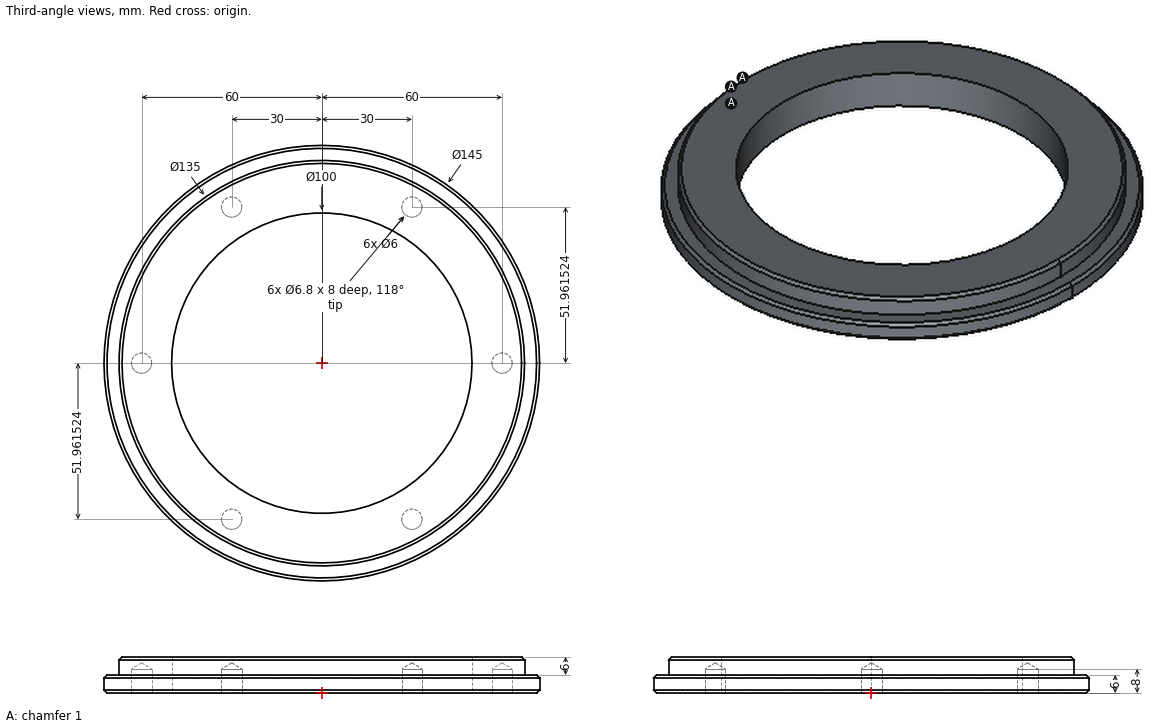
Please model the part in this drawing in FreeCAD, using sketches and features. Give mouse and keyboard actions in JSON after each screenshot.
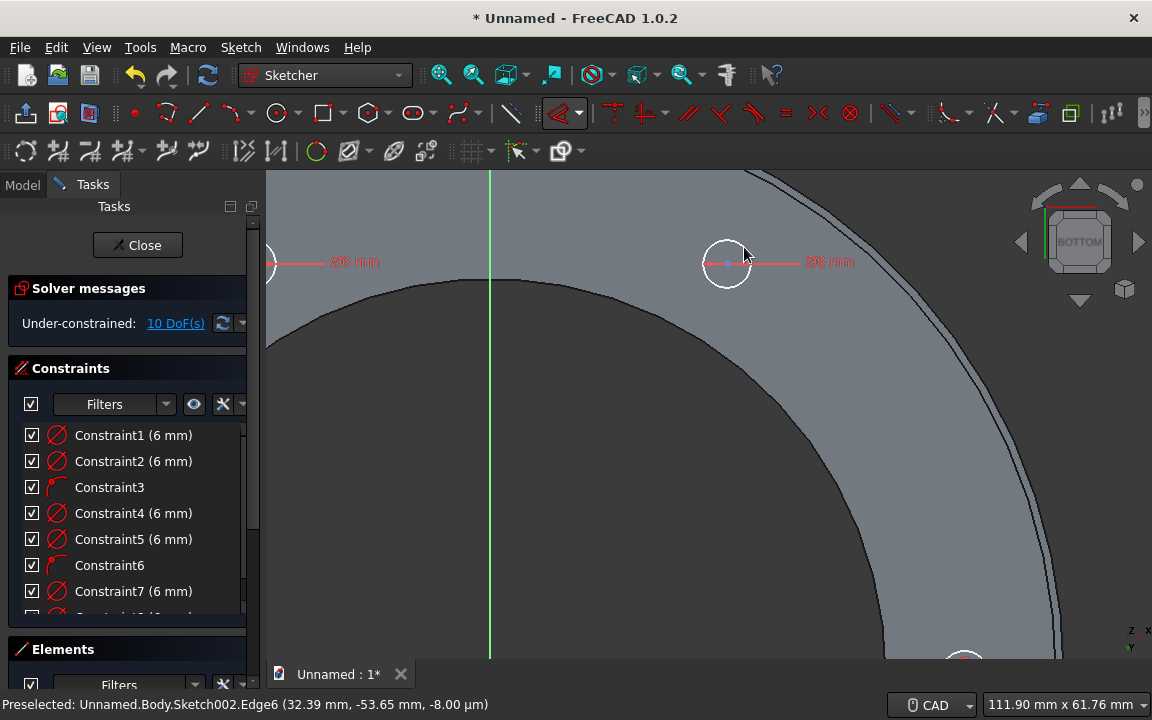
{"action": "scroll", "coordinate": [728, 263], "scroll_direction": "down", "scroll_amount": 5}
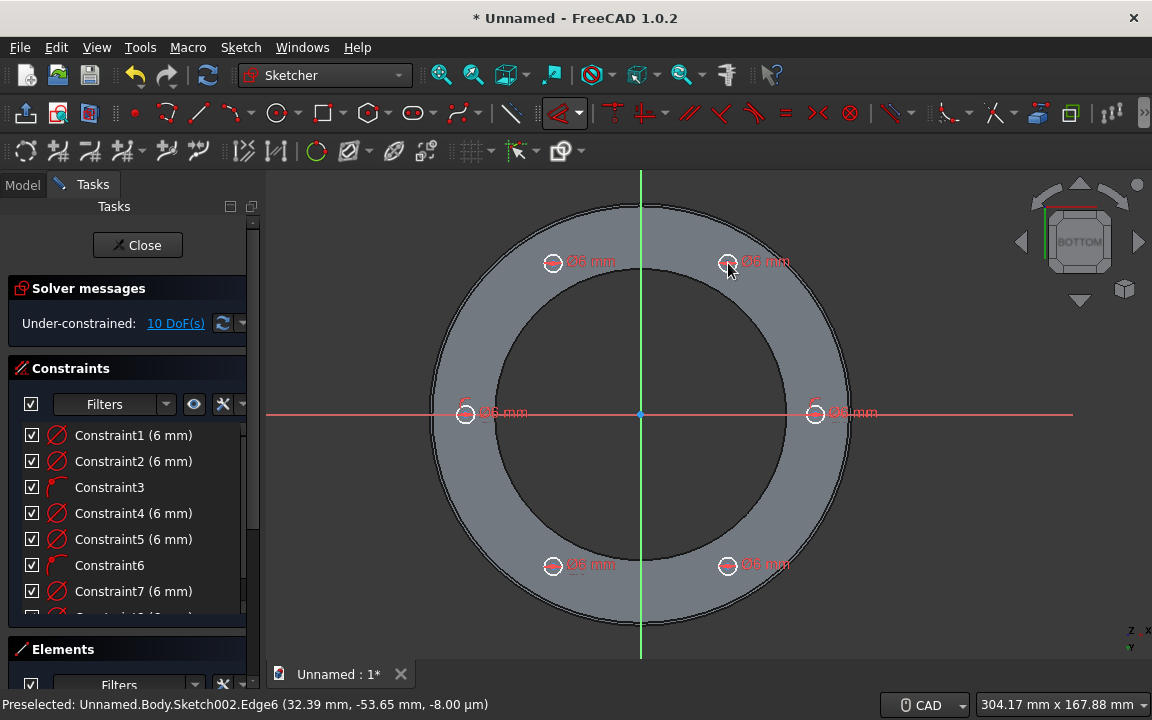
{"action": "left_click", "coordinate": [728, 566]}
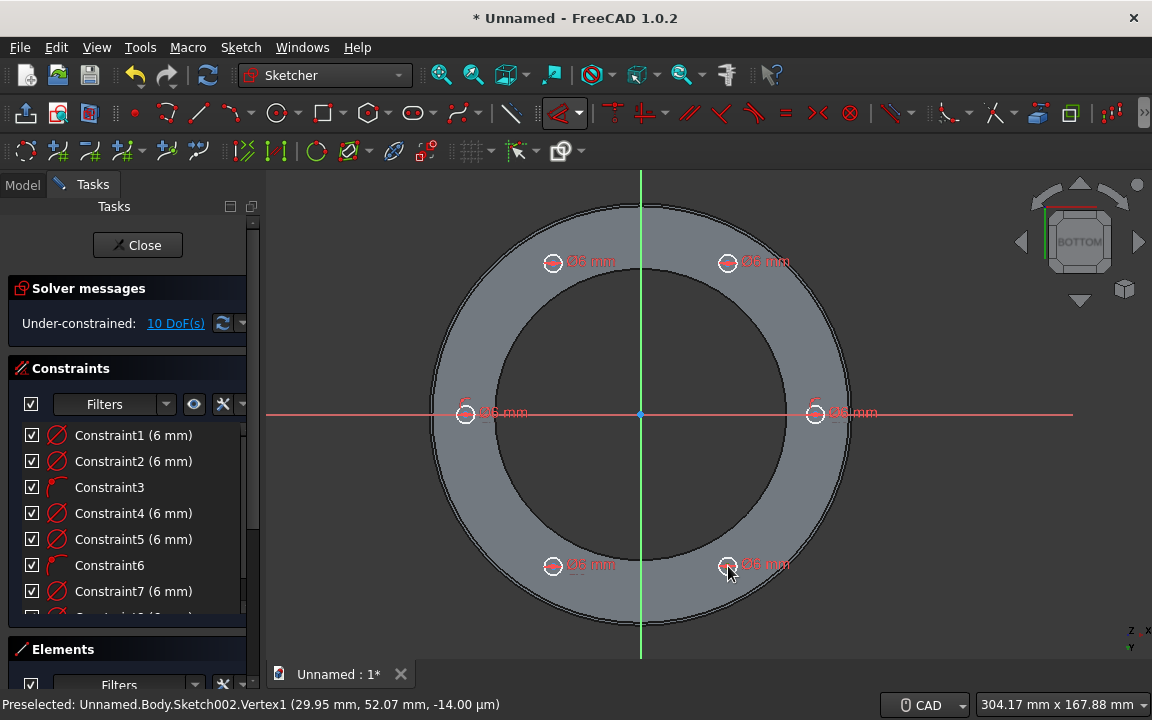
{"action": "left_click", "coordinate": [553, 567]}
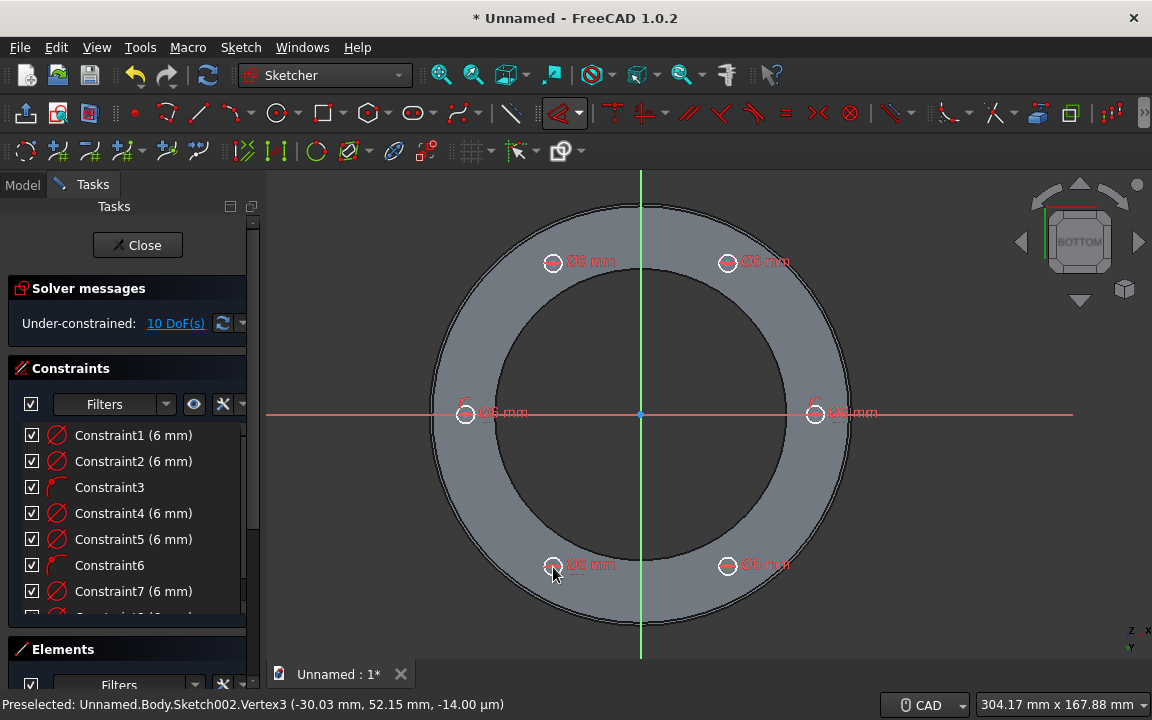
{"action": "left_click", "coordinate": [668, 114]}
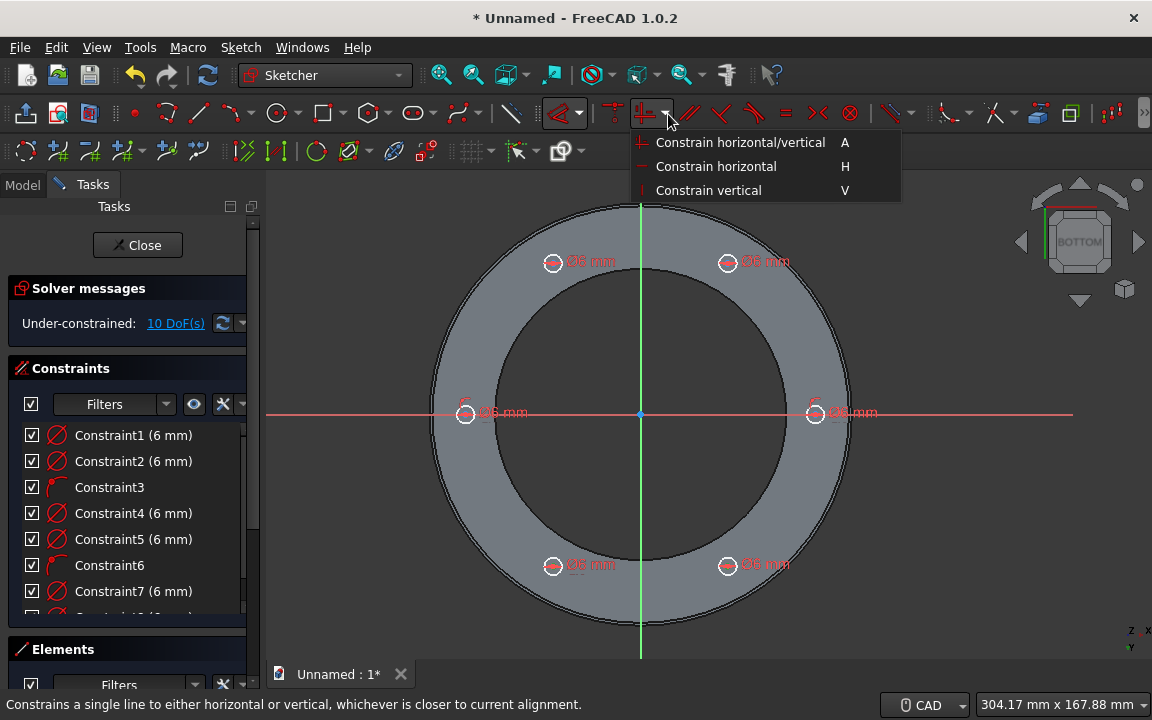
{"action": "left_click", "coordinate": [766, 166]}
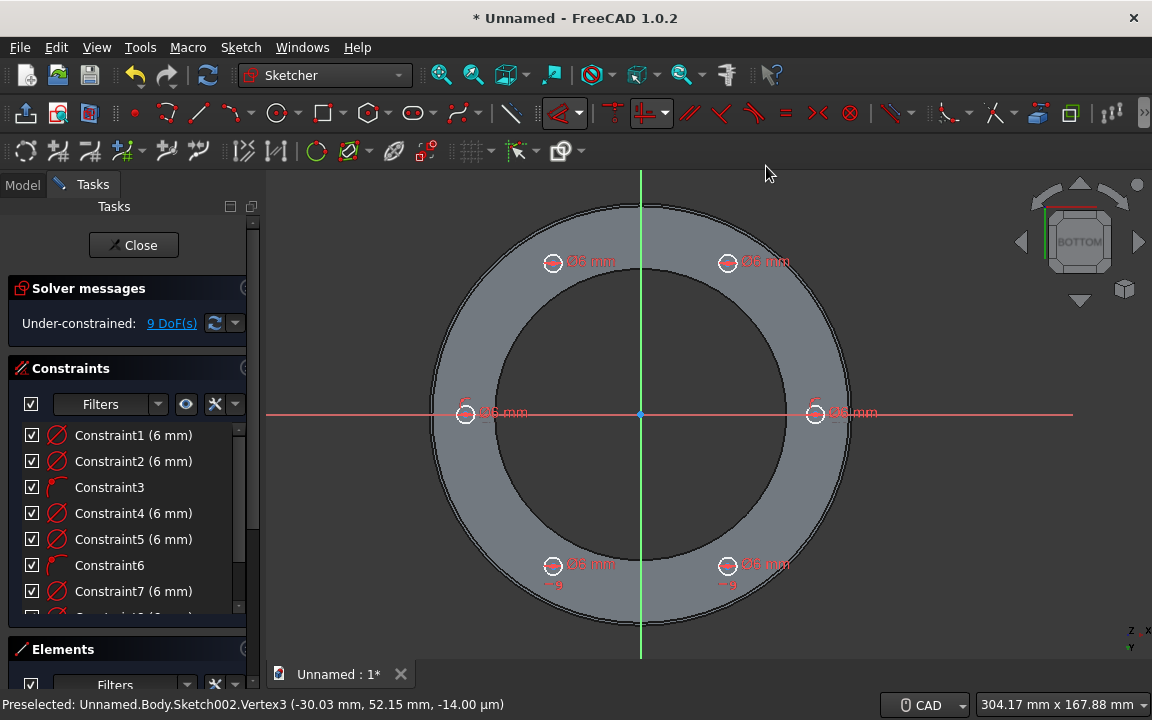
{"action": "left_click", "coordinate": [553, 566]}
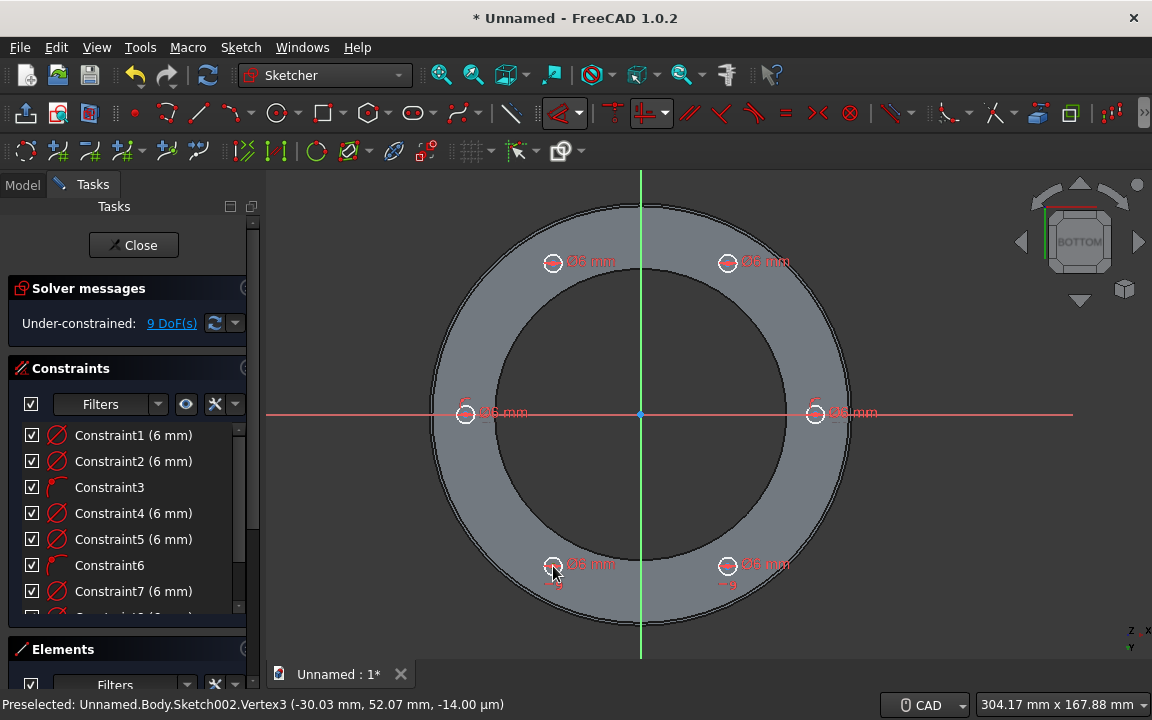
{"action": "left_click", "coordinate": [553, 263]}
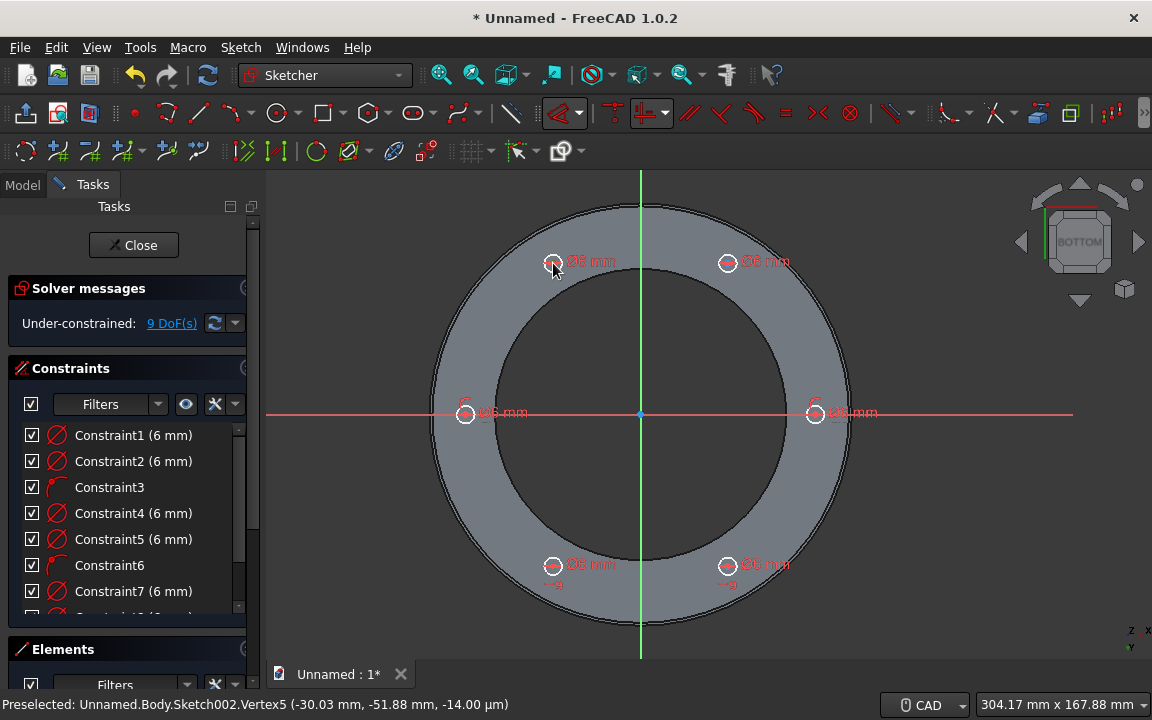
{"action": "left_click", "coordinate": [668, 114]}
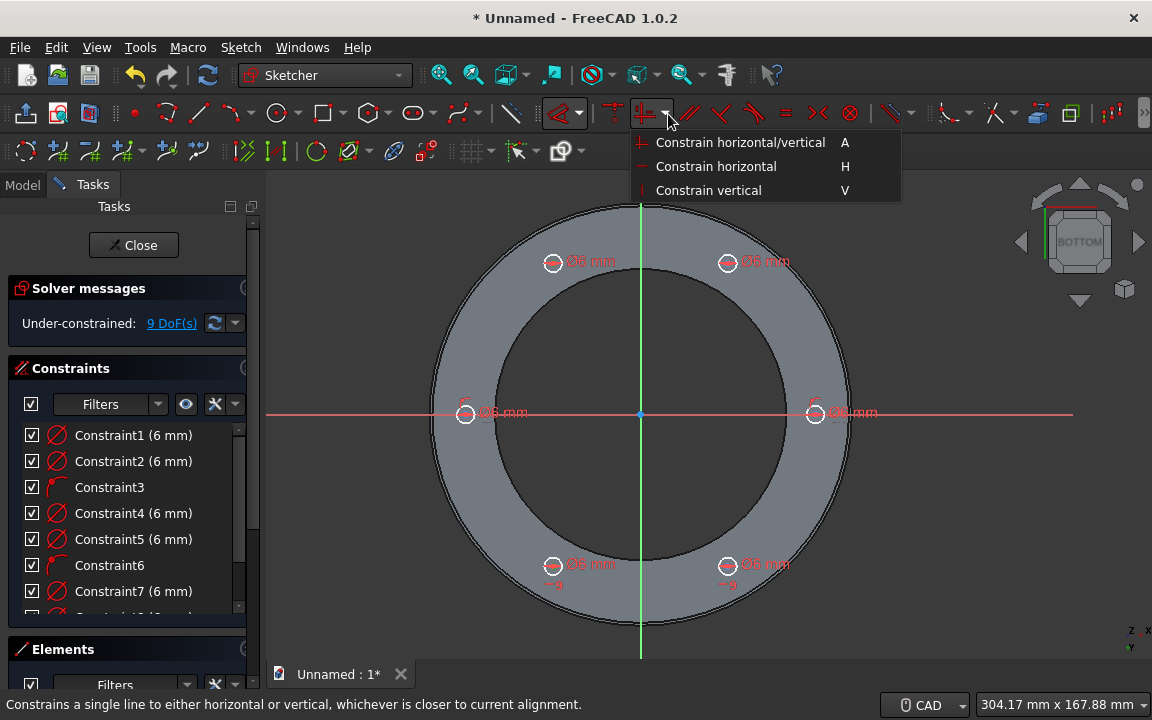
{"action": "left_click", "coordinate": [766, 190]}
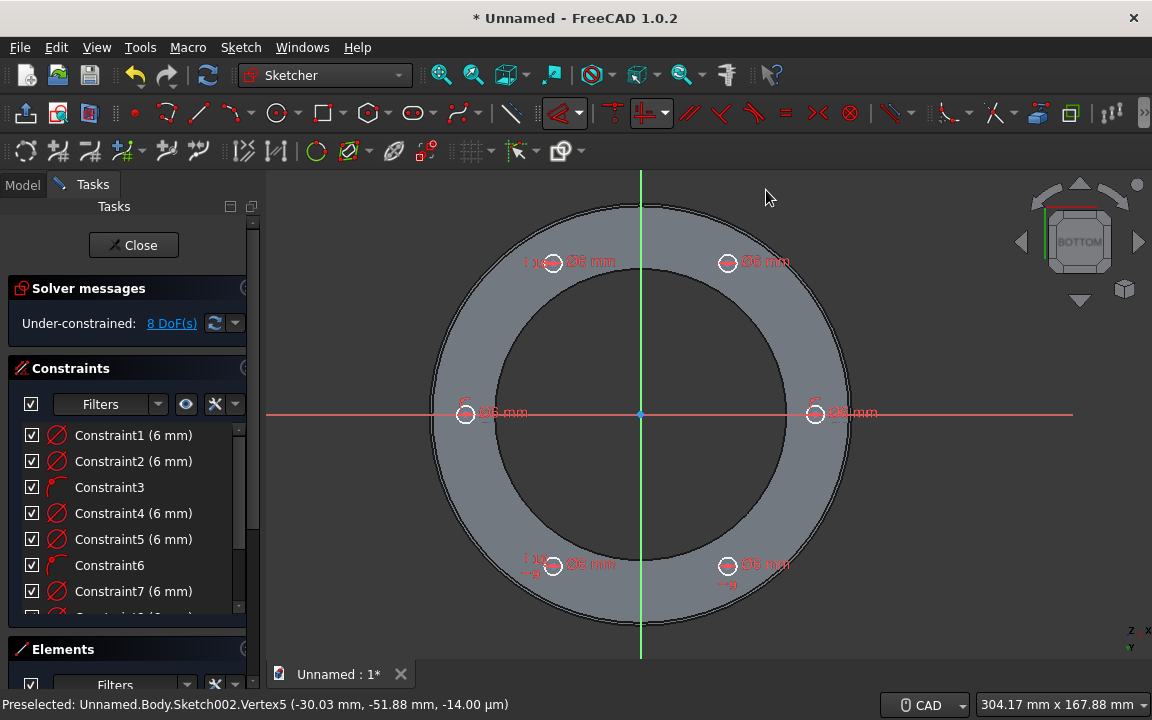
{"action": "left_click", "coordinate": [728, 566]}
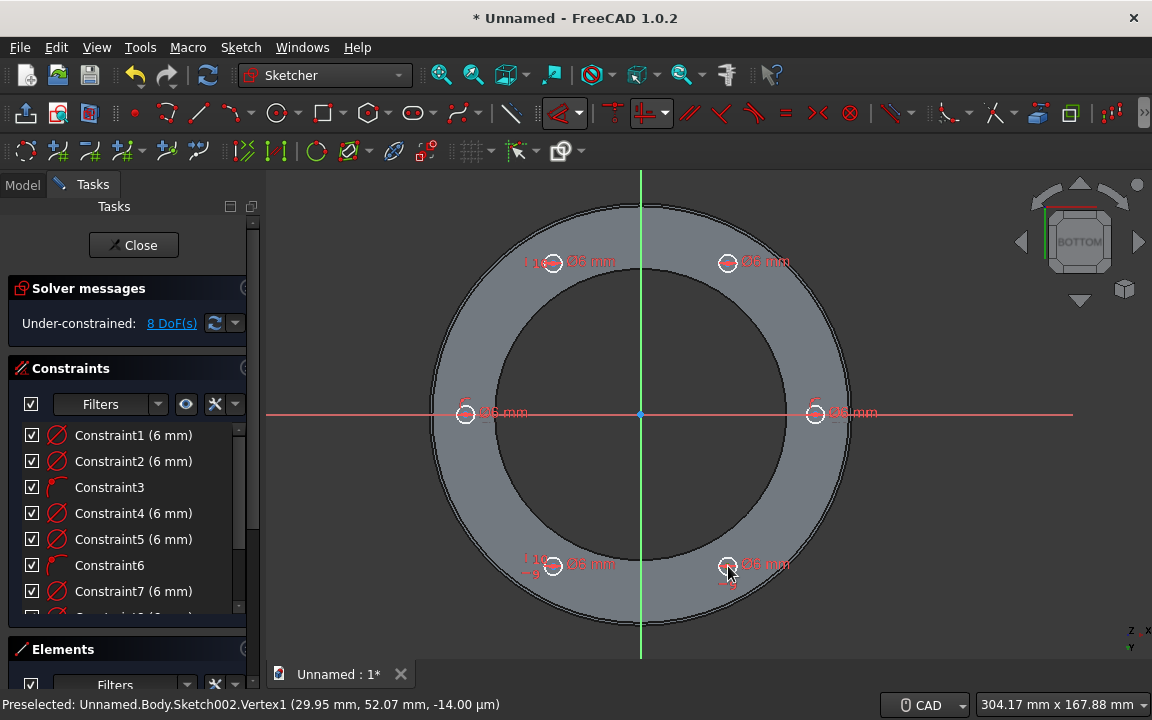
{"action": "left_click", "coordinate": [728, 263]}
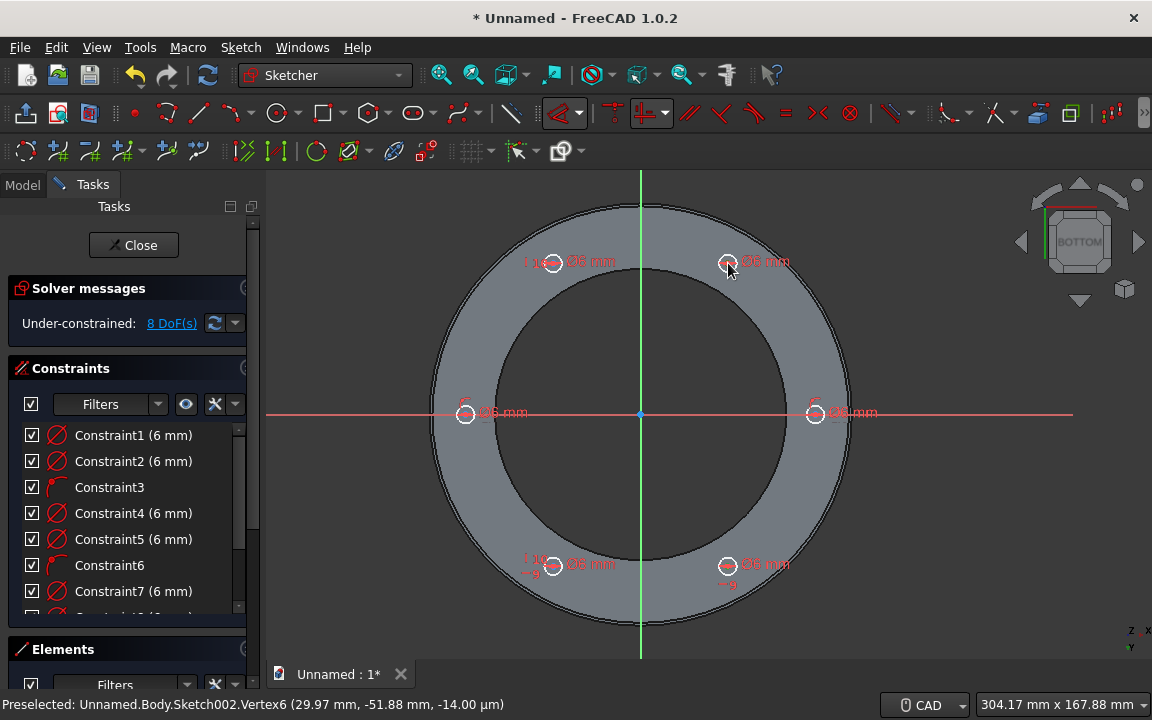
{"action": "left_click", "coordinate": [668, 114]}